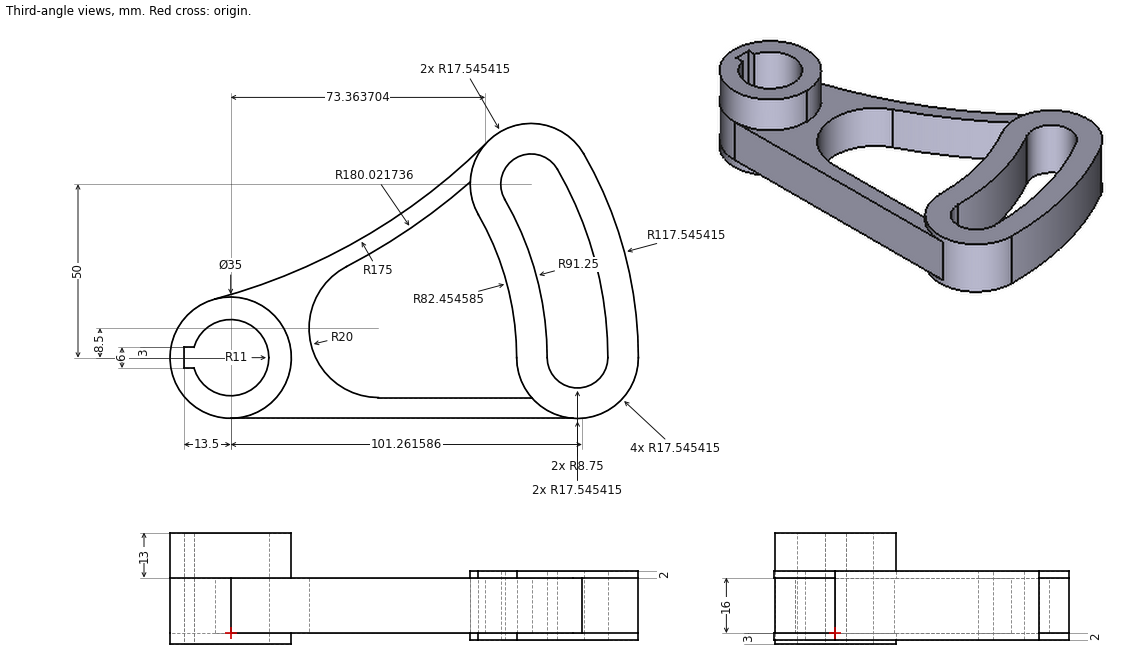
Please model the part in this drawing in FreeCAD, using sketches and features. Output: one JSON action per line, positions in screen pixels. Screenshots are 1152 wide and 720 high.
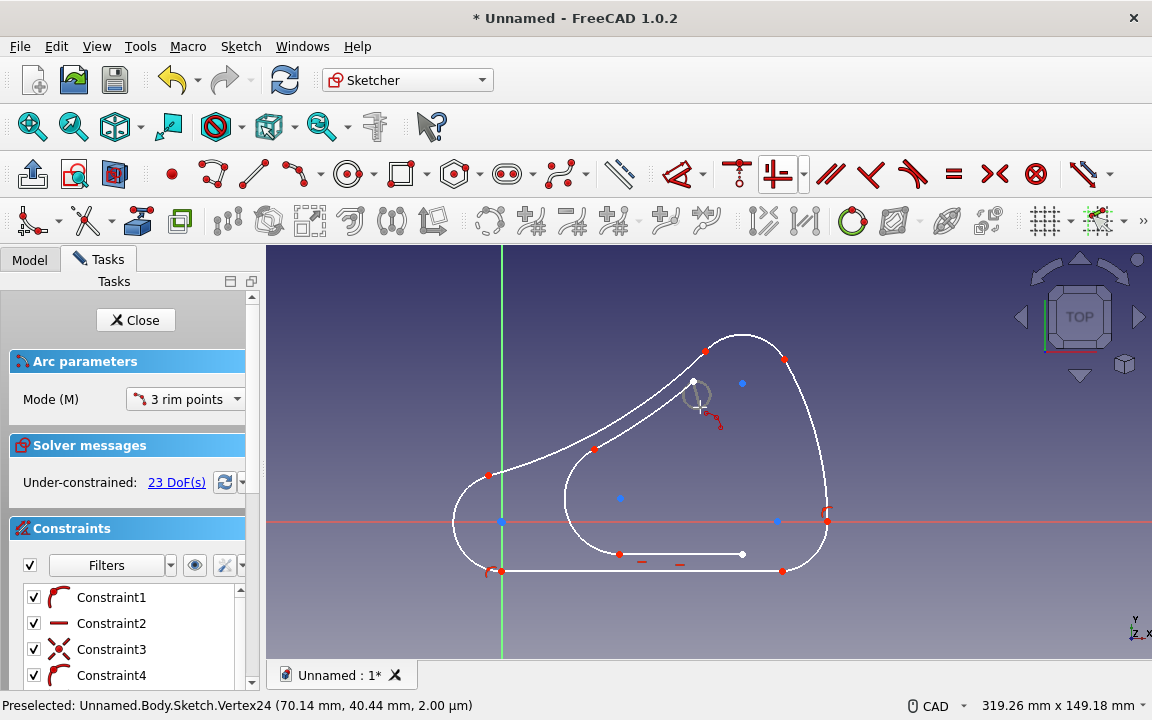
{"action": "scroll", "coordinate": [695, 395], "scroll_direction": "up", "scroll_amount": 11}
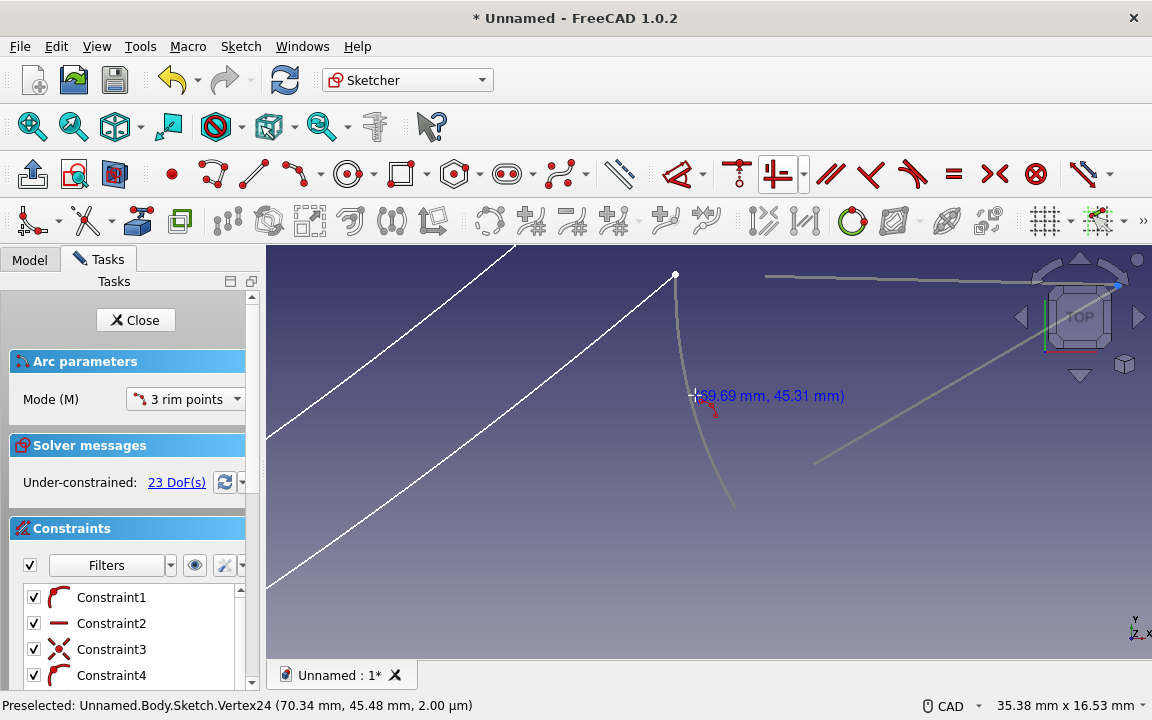
{"action": "left_click", "coordinate": [688, 389]}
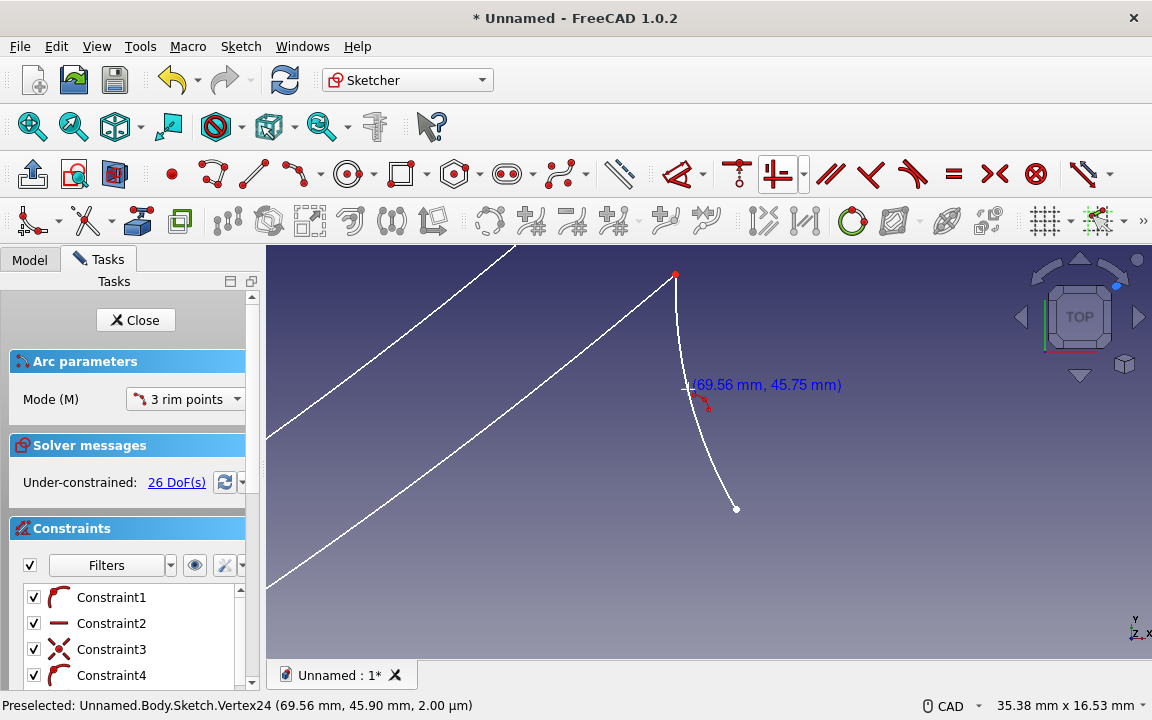
{"action": "scroll", "coordinate": [695, 395], "scroll_direction": "down", "scroll_amount": 11}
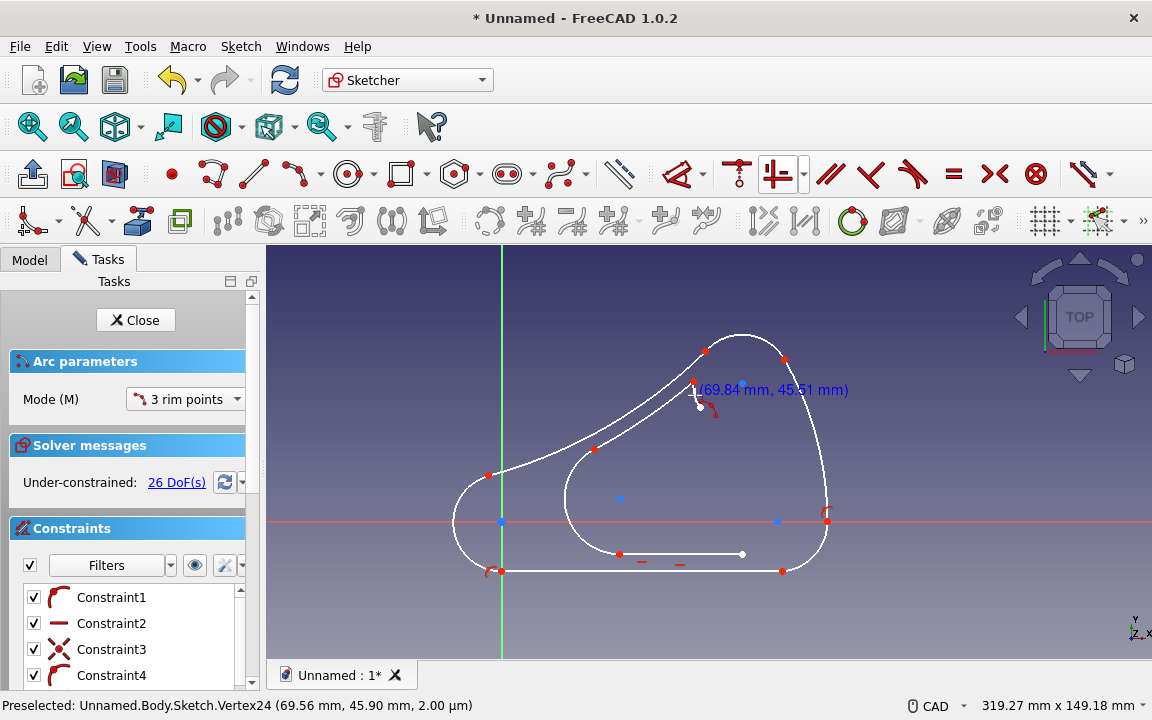
{"action": "left_click", "coordinate": [700, 408]}
{"action": "left_click", "coordinate": [730, 522]}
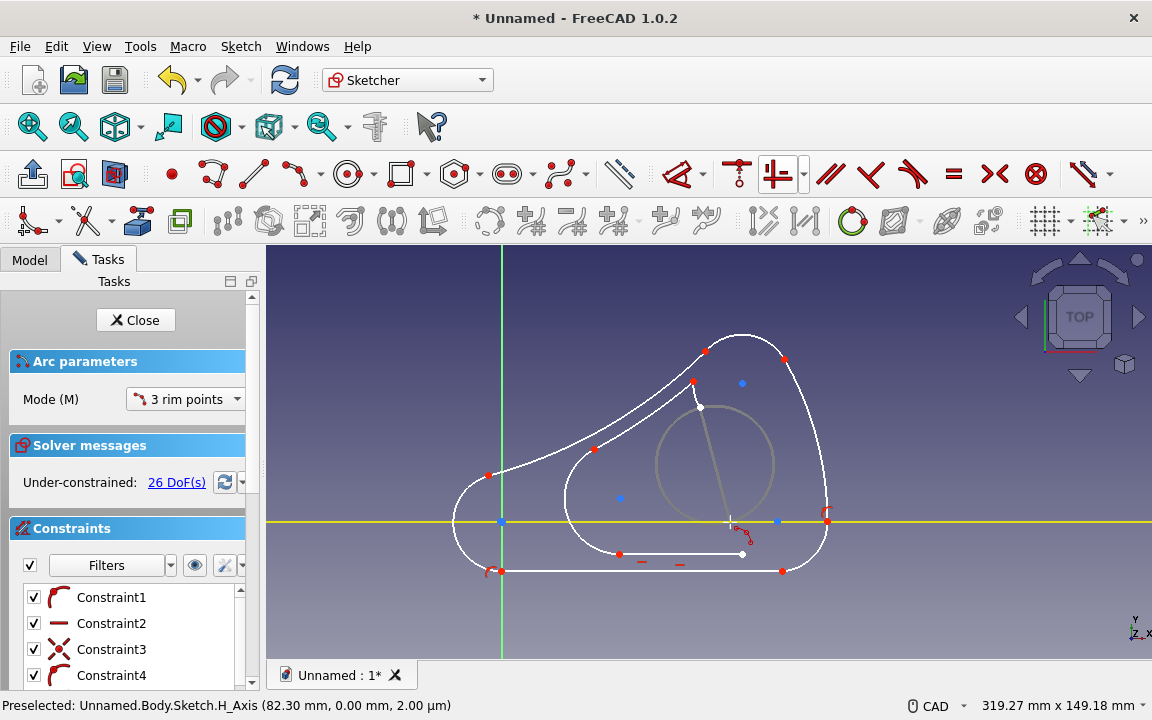
{"action": "scroll", "coordinate": [723, 463], "scroll_direction": "up", "scroll_amount": 4}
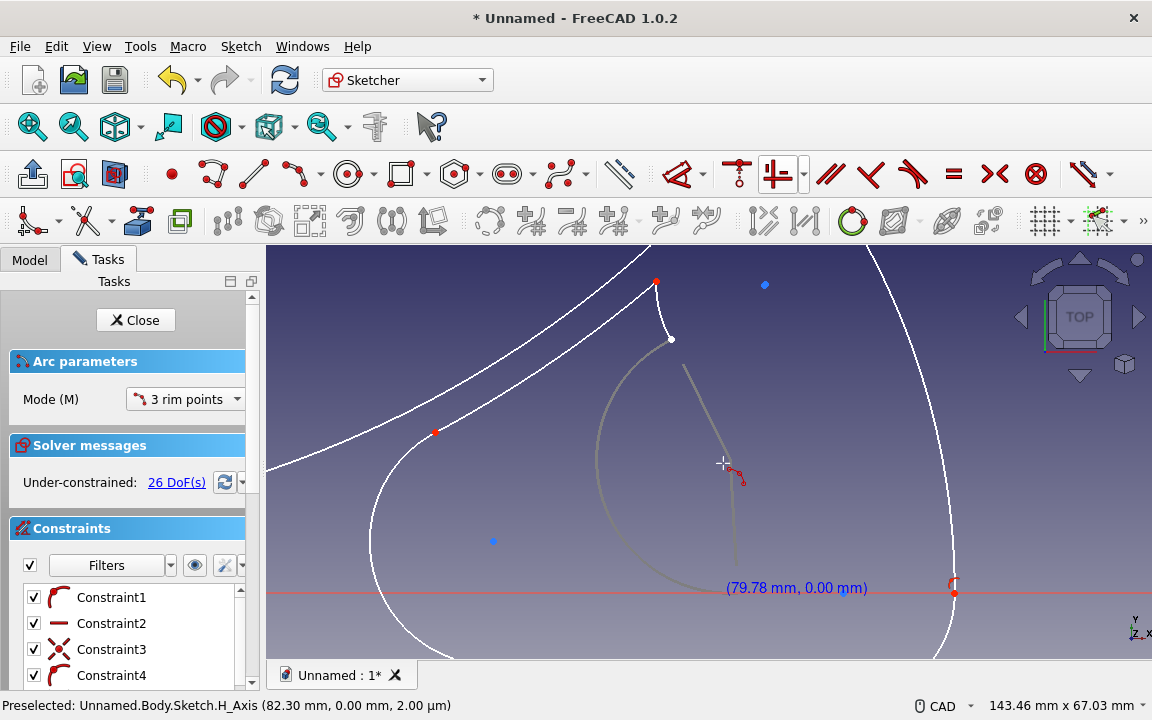
{"action": "left_click", "coordinate": [722, 461]}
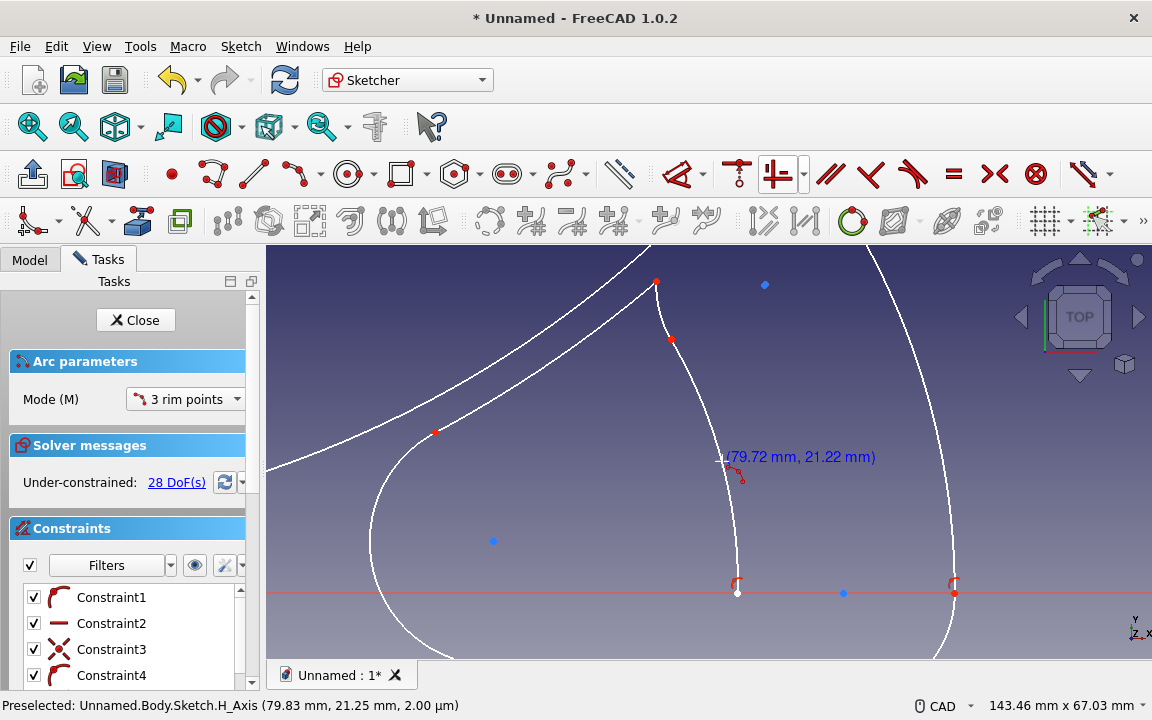
{"action": "left_click", "coordinate": [738, 593]}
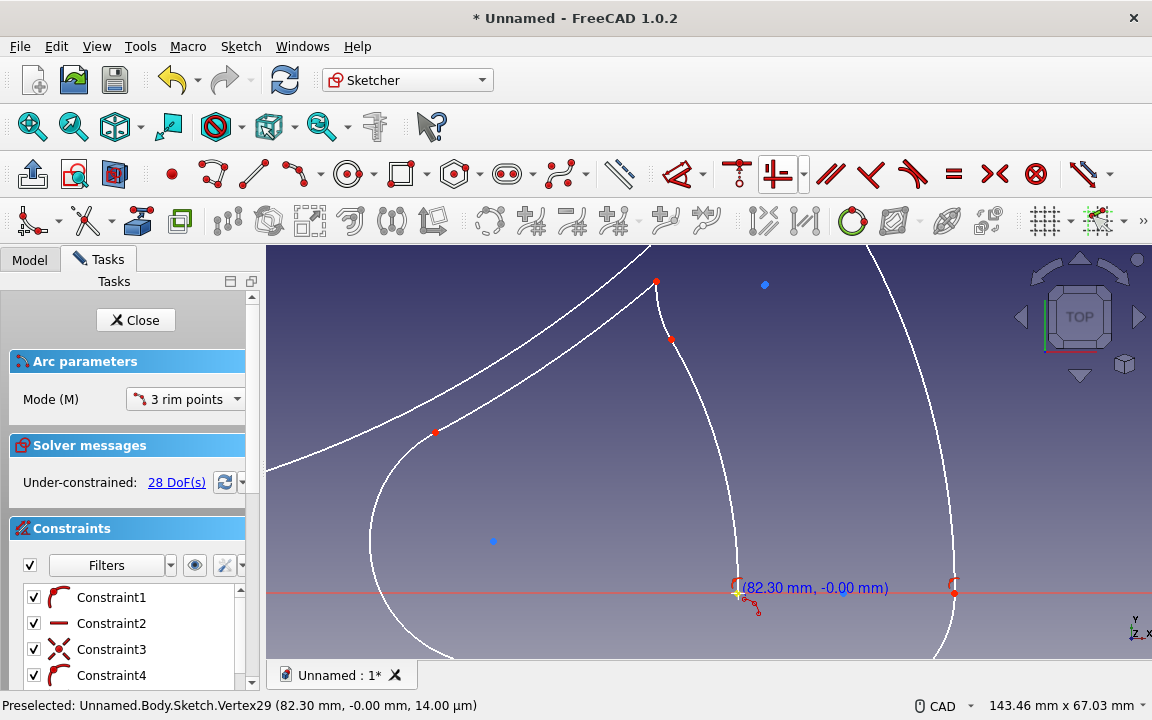
{"action": "scroll", "coordinate": [723, 463], "scroll_direction": "down", "scroll_amount": 4}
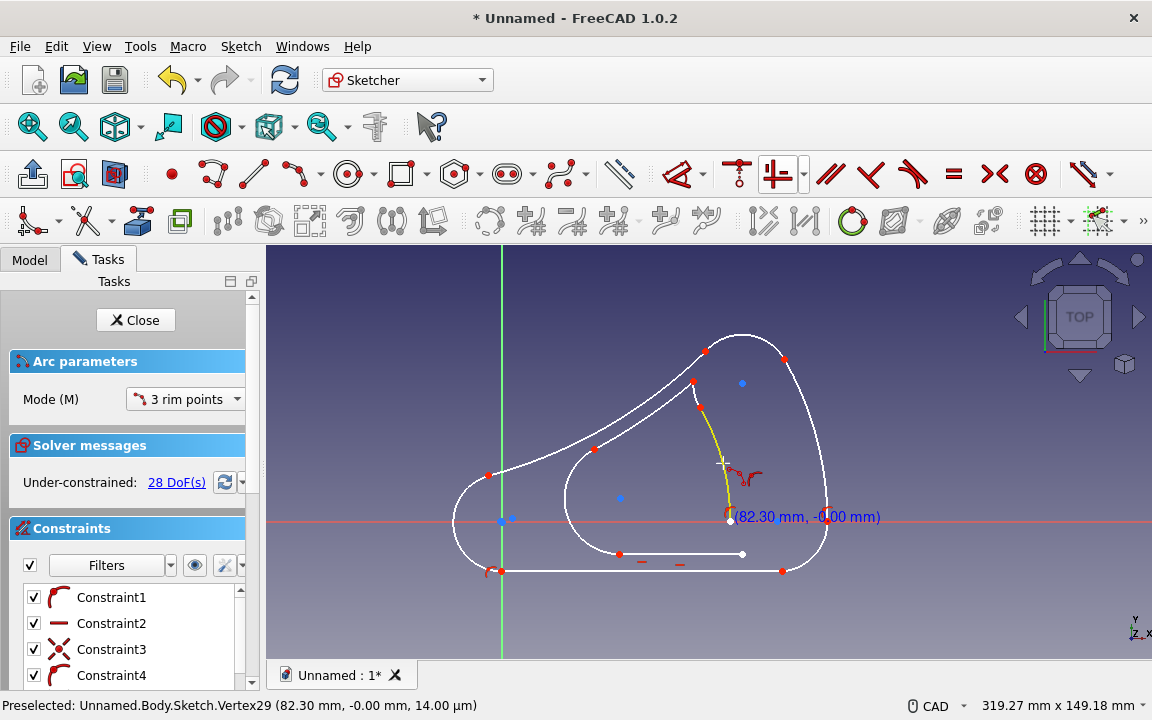
{"action": "left_click", "coordinate": [742, 554]}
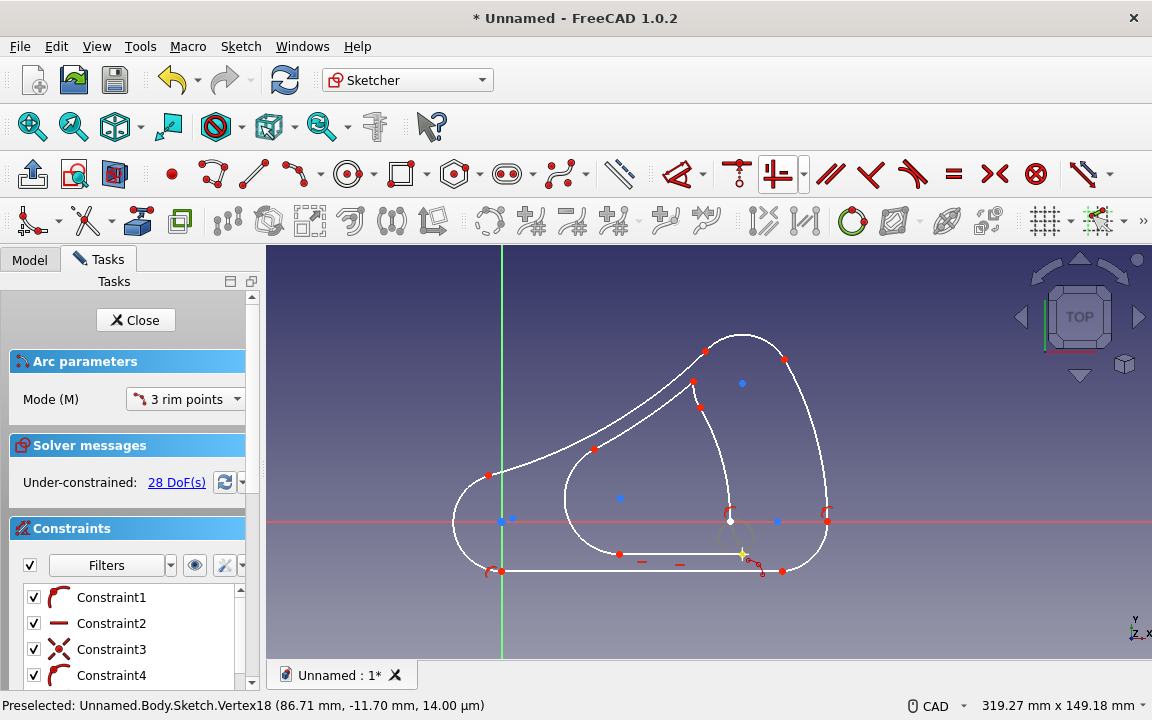
{"action": "scroll", "coordinate": [734, 539], "scroll_direction": "up", "scroll_amount": 9}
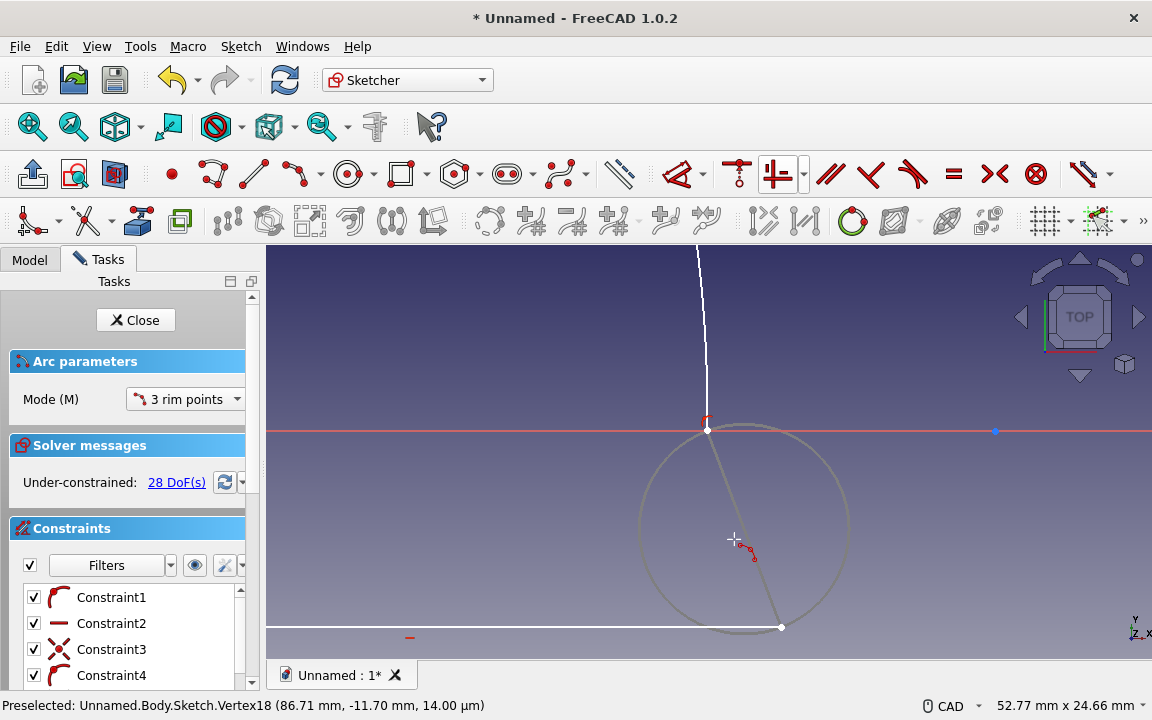
{"action": "left_click", "coordinate": [728, 534]}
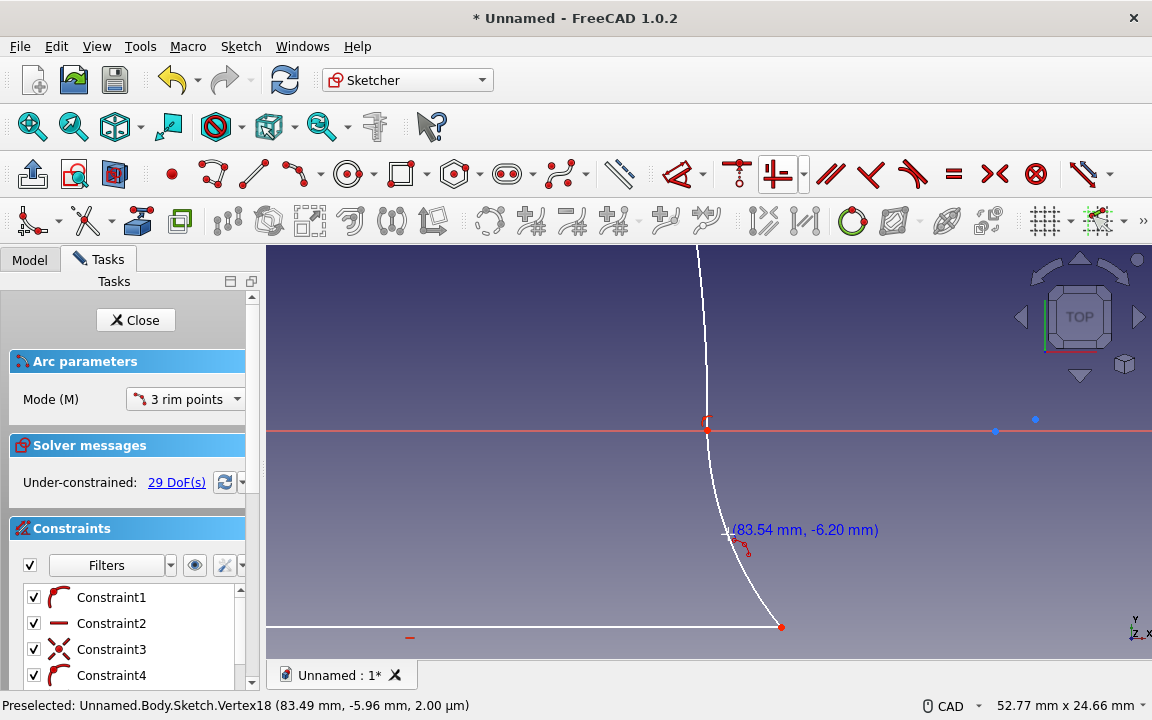
{"action": "scroll", "coordinate": [734, 539], "scroll_direction": "down", "scroll_amount": 9}